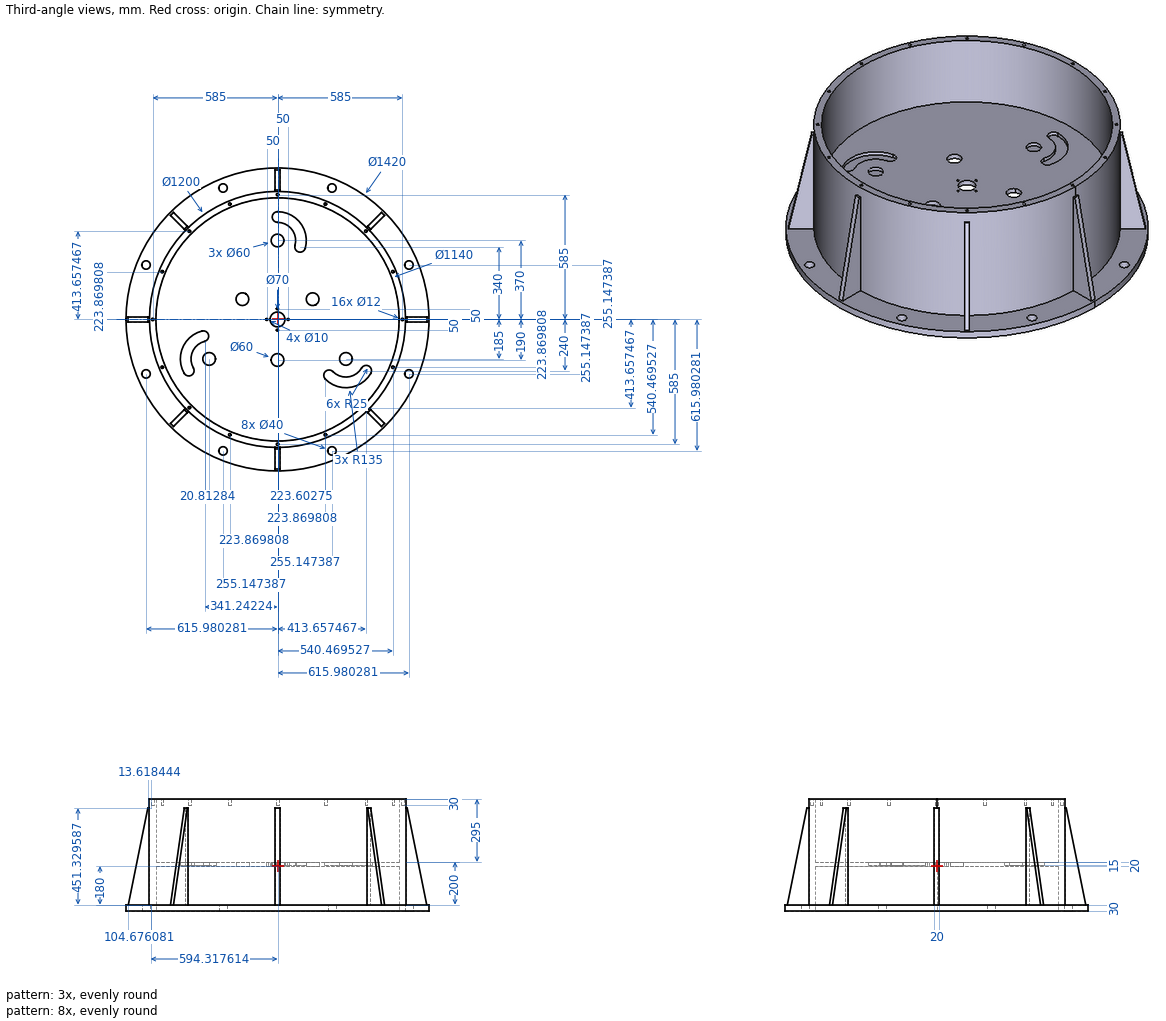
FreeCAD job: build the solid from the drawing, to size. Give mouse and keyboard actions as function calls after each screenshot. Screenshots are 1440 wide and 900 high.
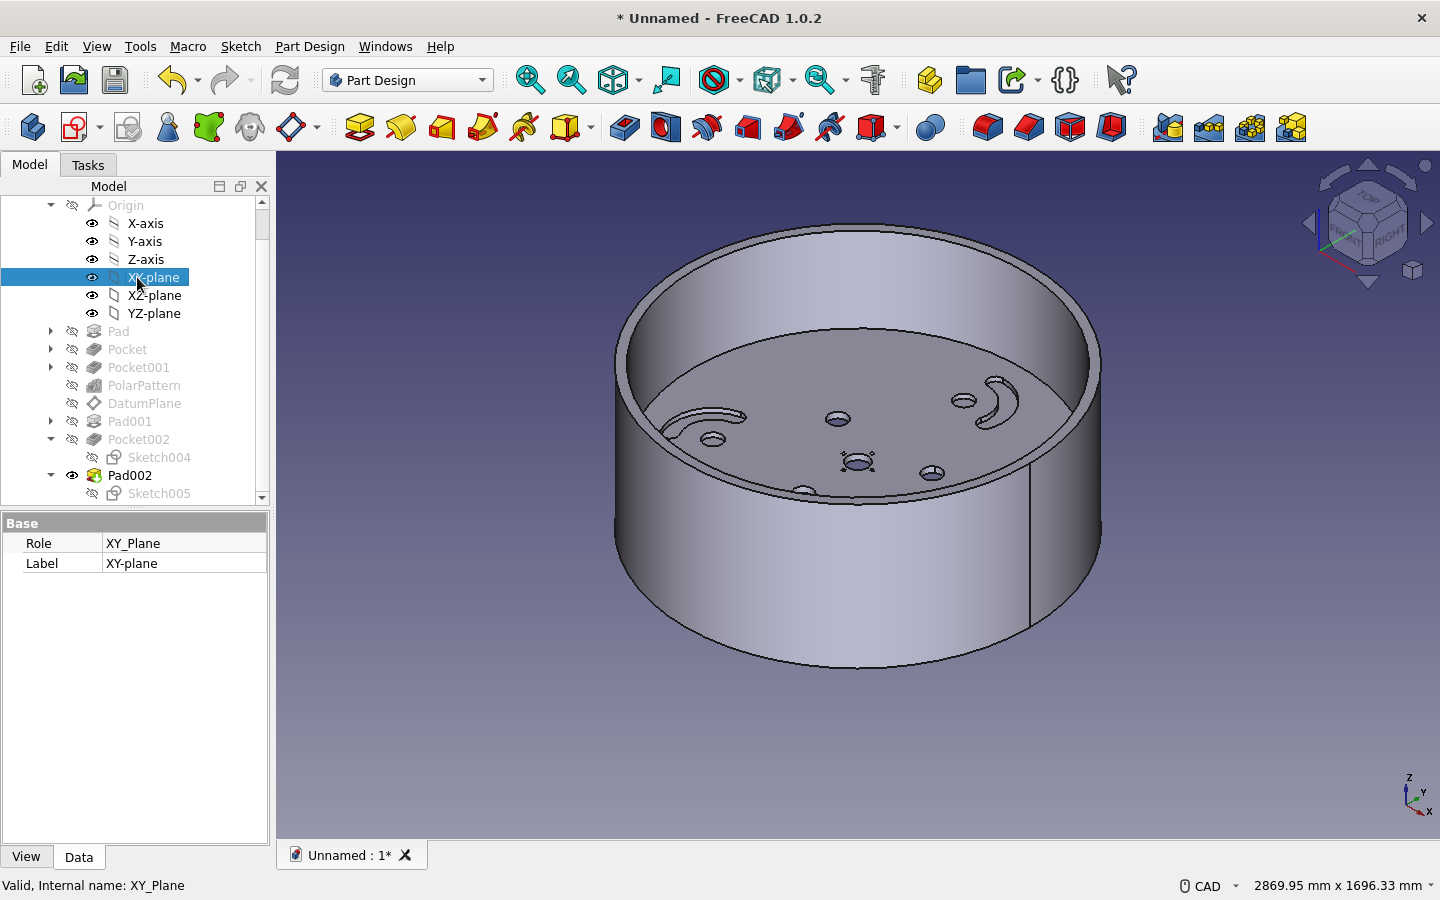
click(290, 128)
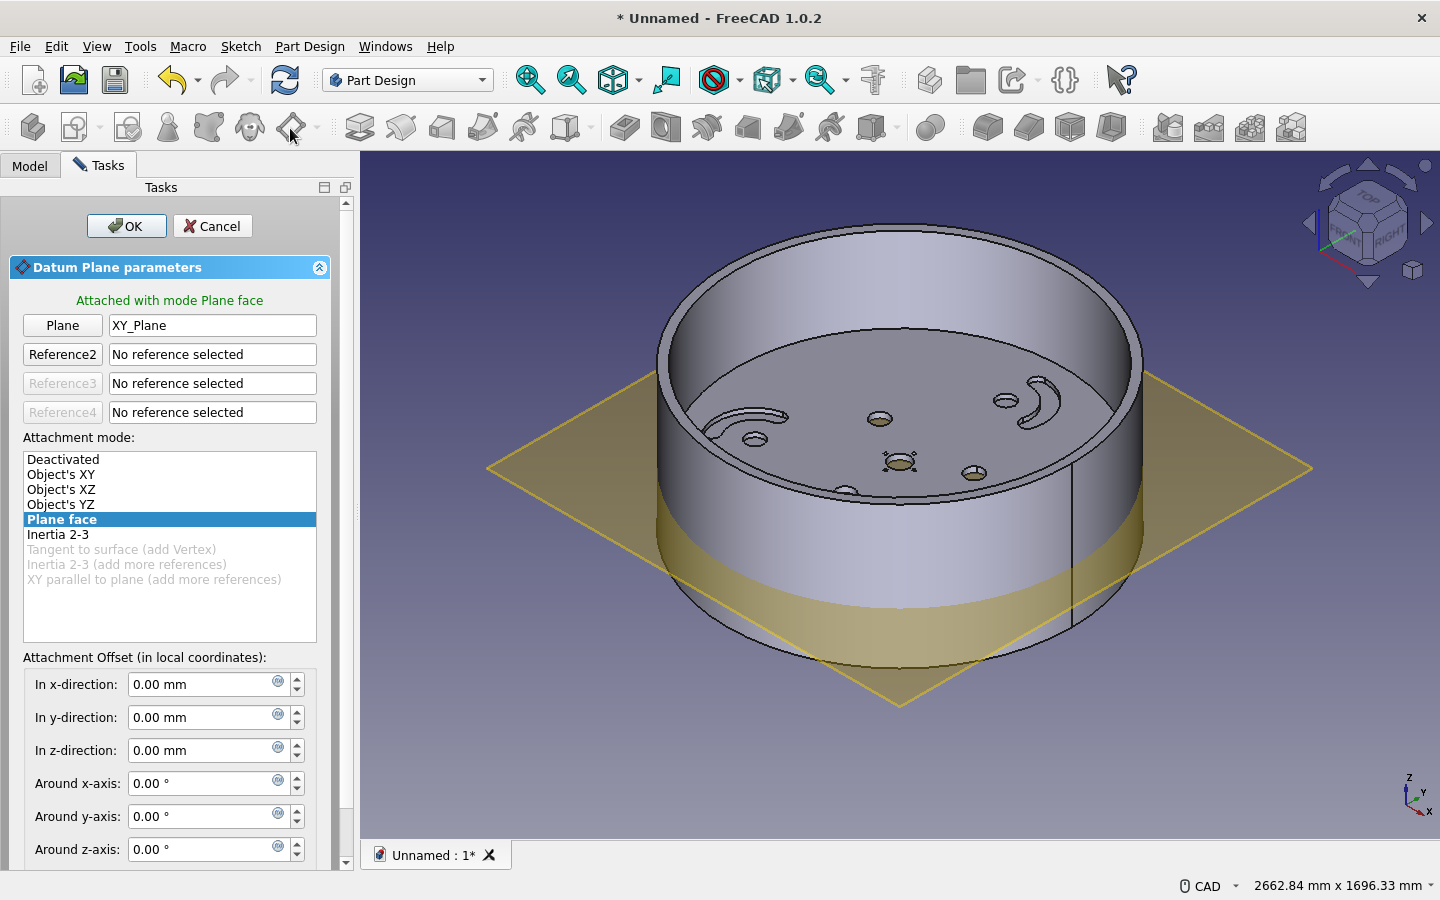
triple_click(210, 750)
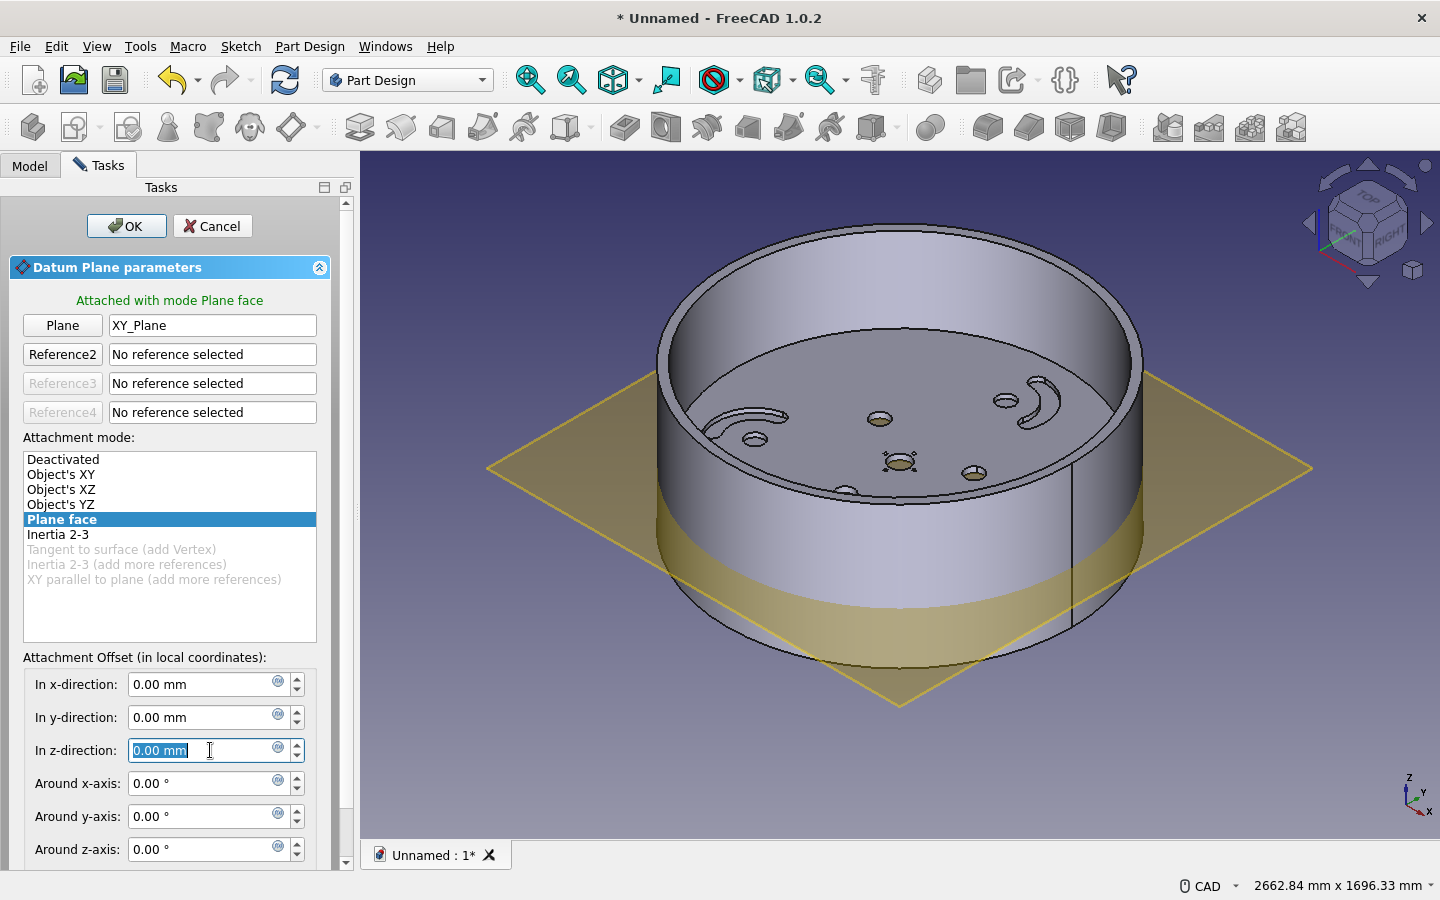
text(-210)
key(Tab)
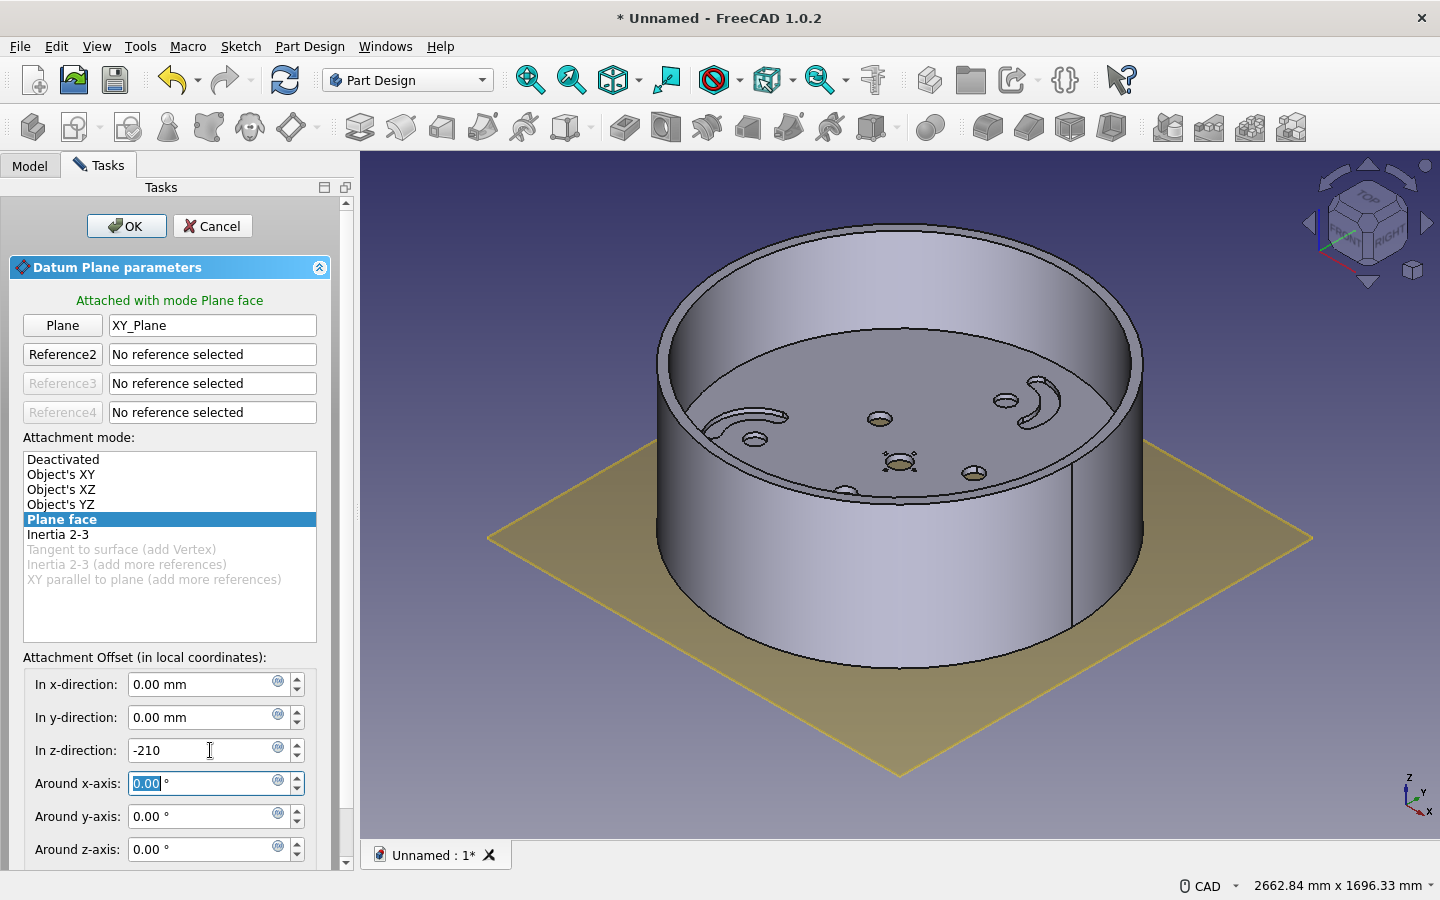
click(127, 226)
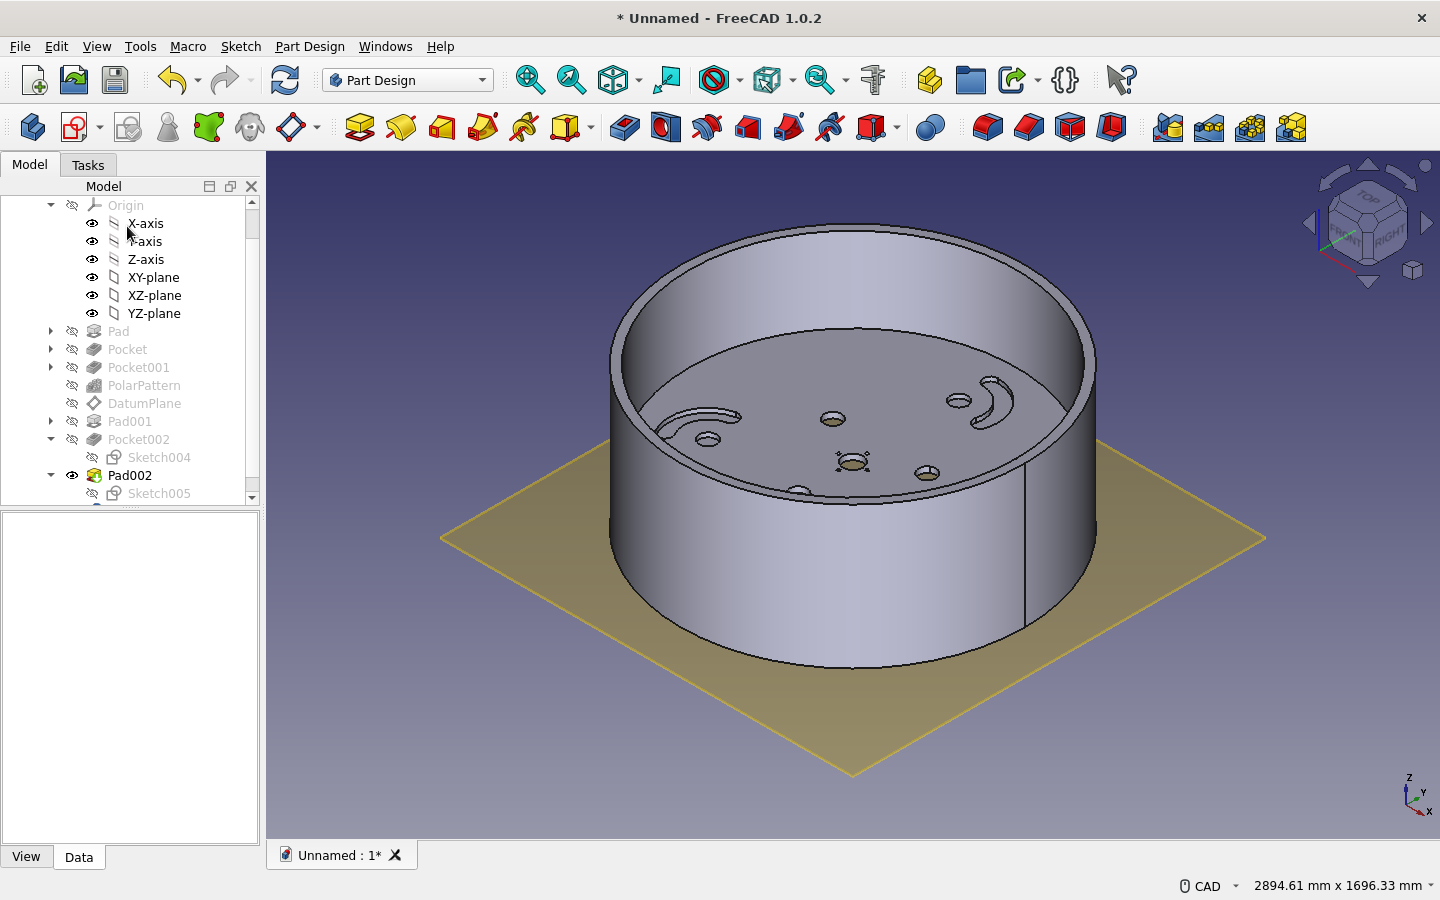
scroll(141, 345, down, 3)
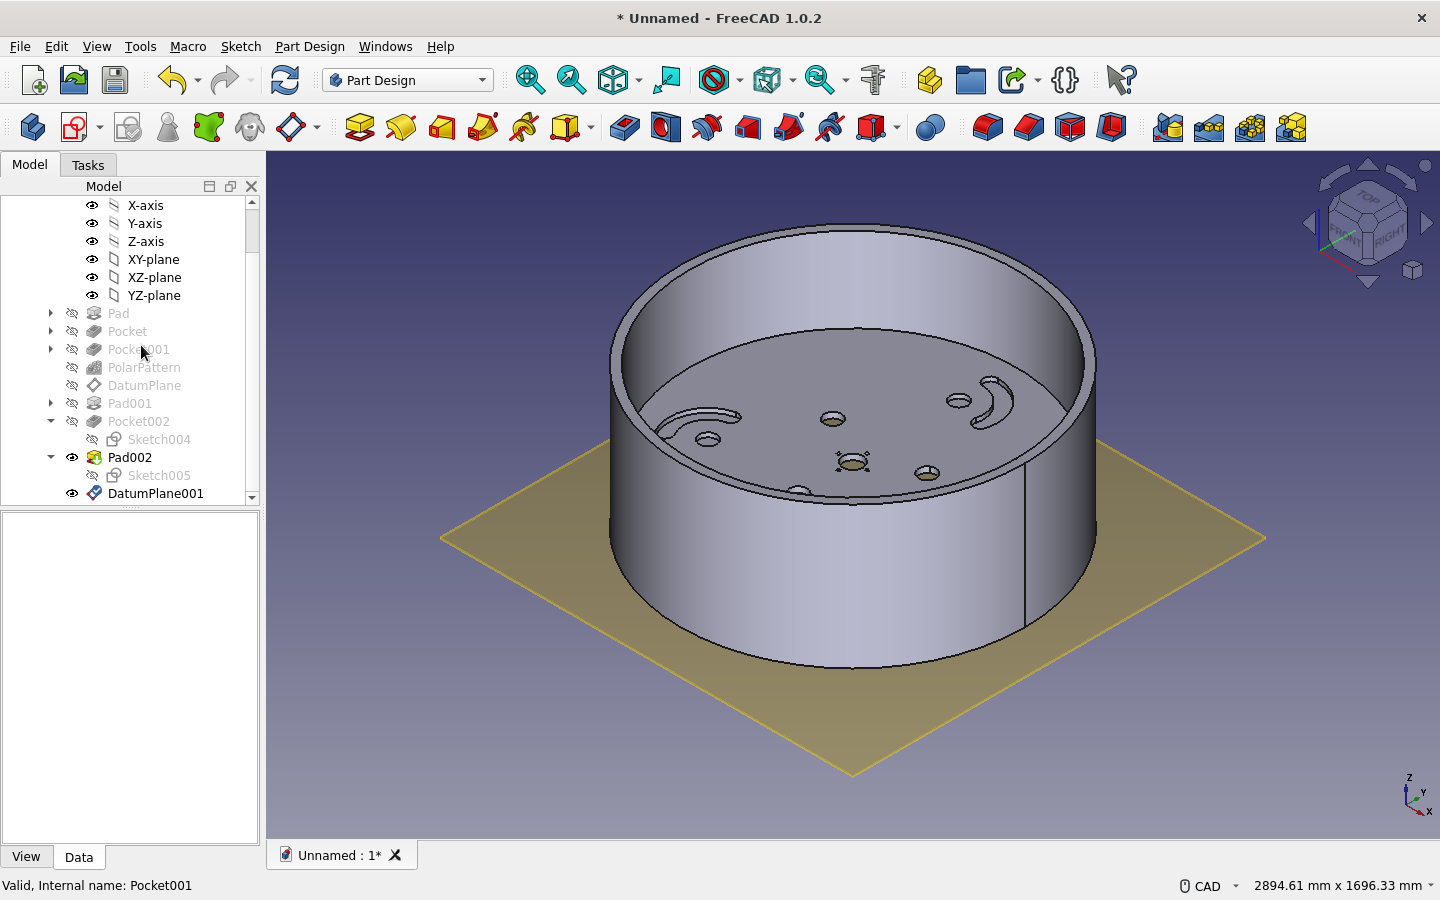
click(117, 493)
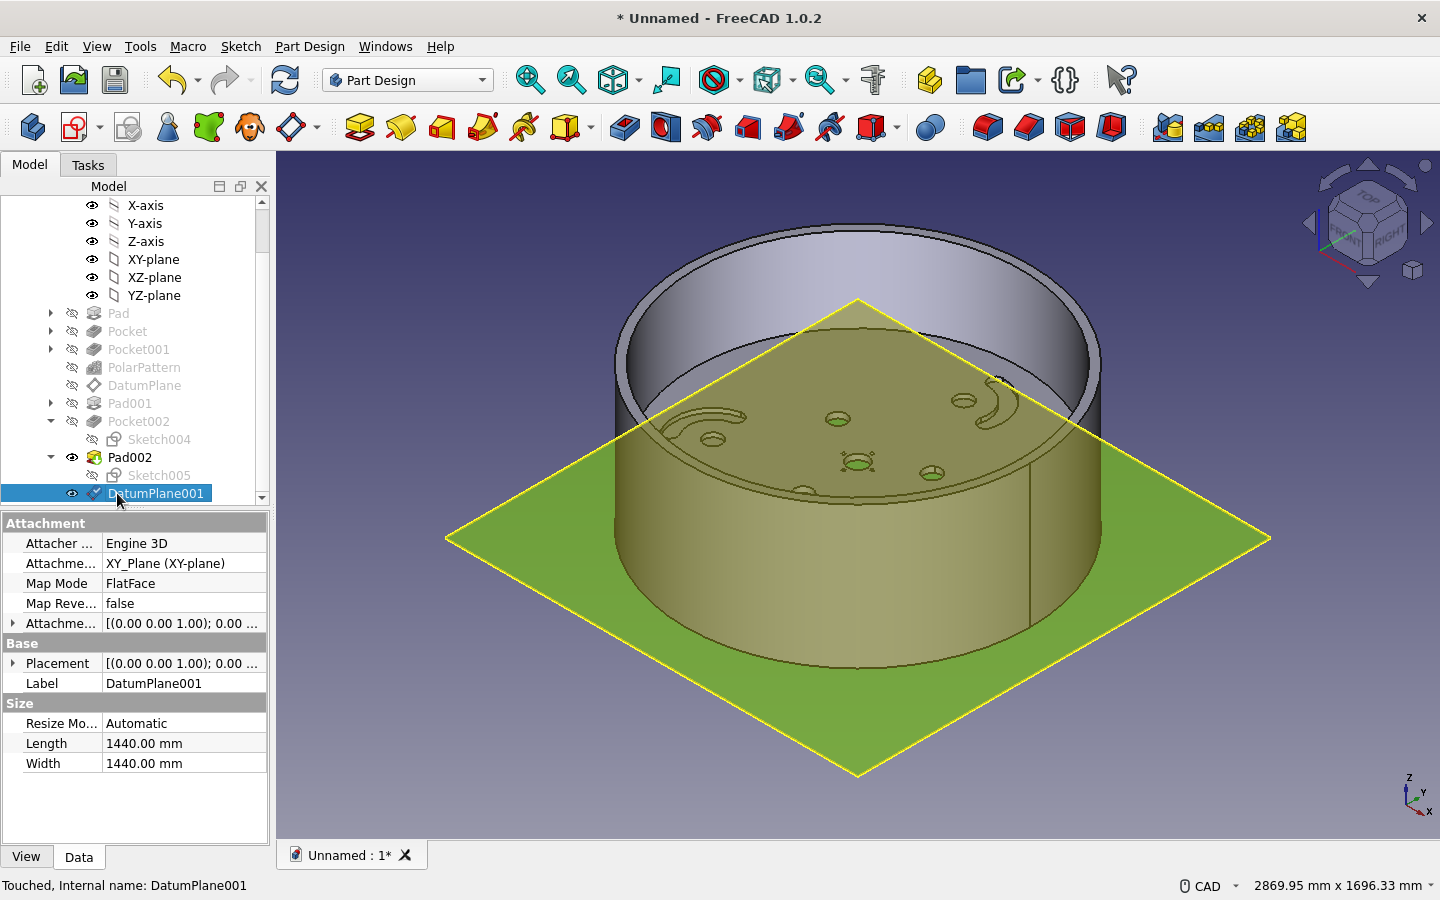
click(74, 128)